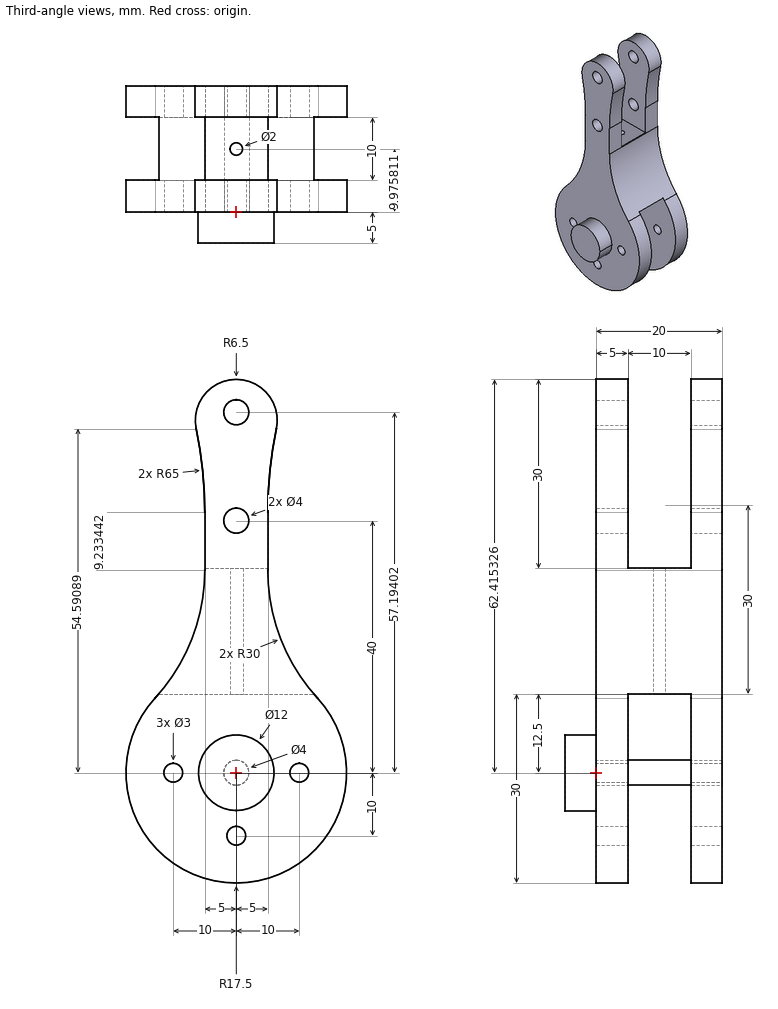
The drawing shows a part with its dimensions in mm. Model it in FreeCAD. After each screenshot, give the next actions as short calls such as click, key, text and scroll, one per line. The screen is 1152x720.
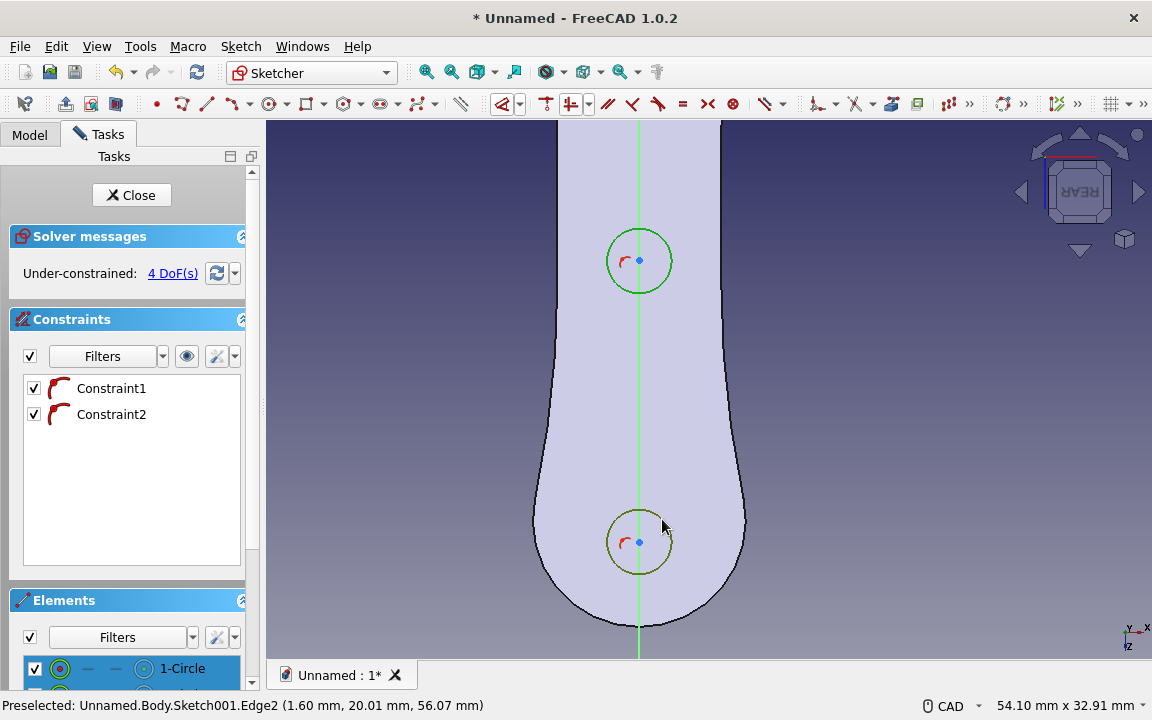
click(683, 104)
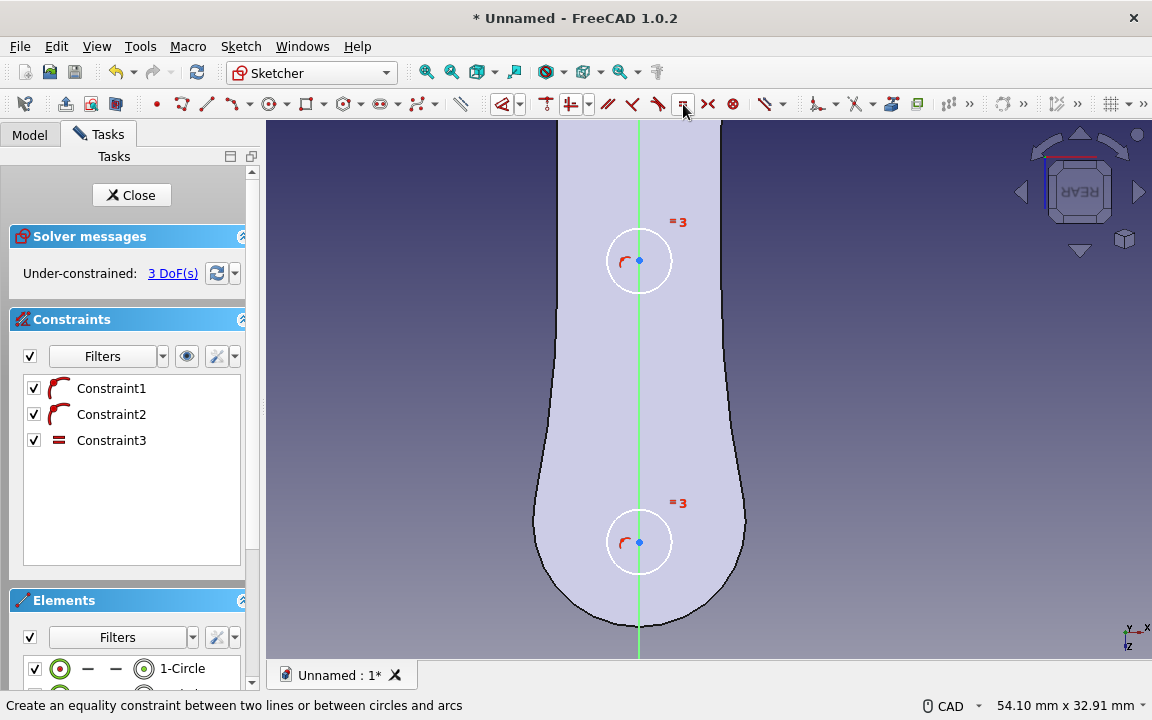
click(662, 238)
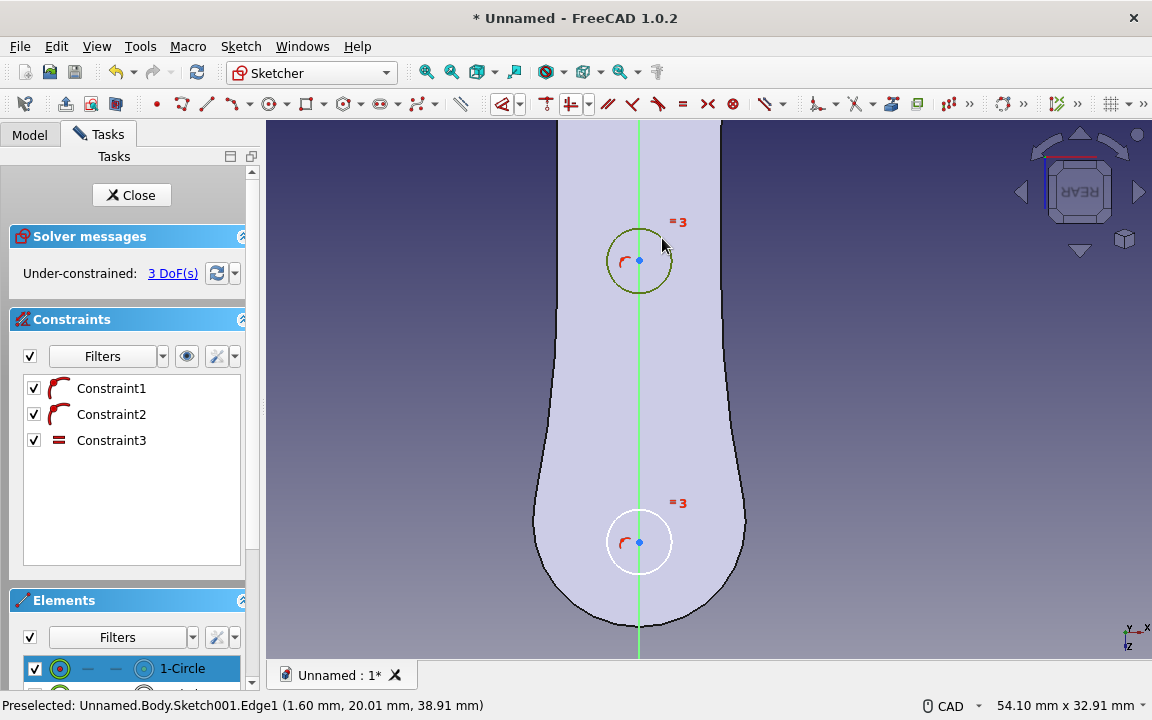
key(k)
key(o)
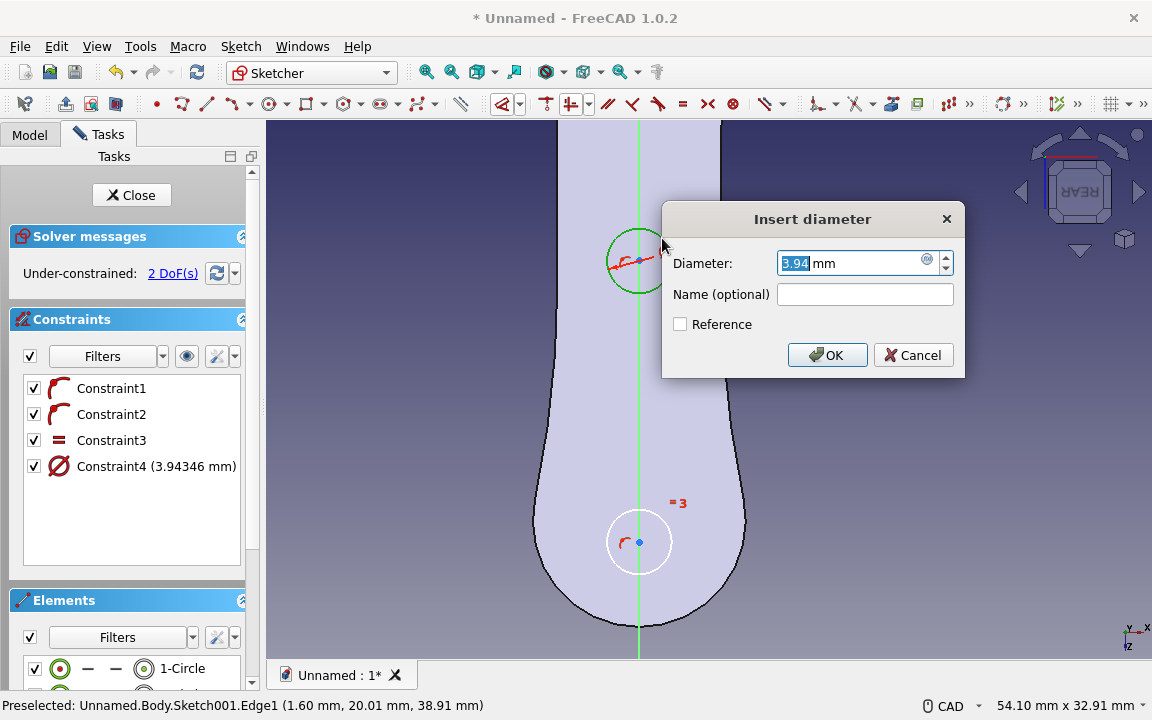
text(4)
key(Return)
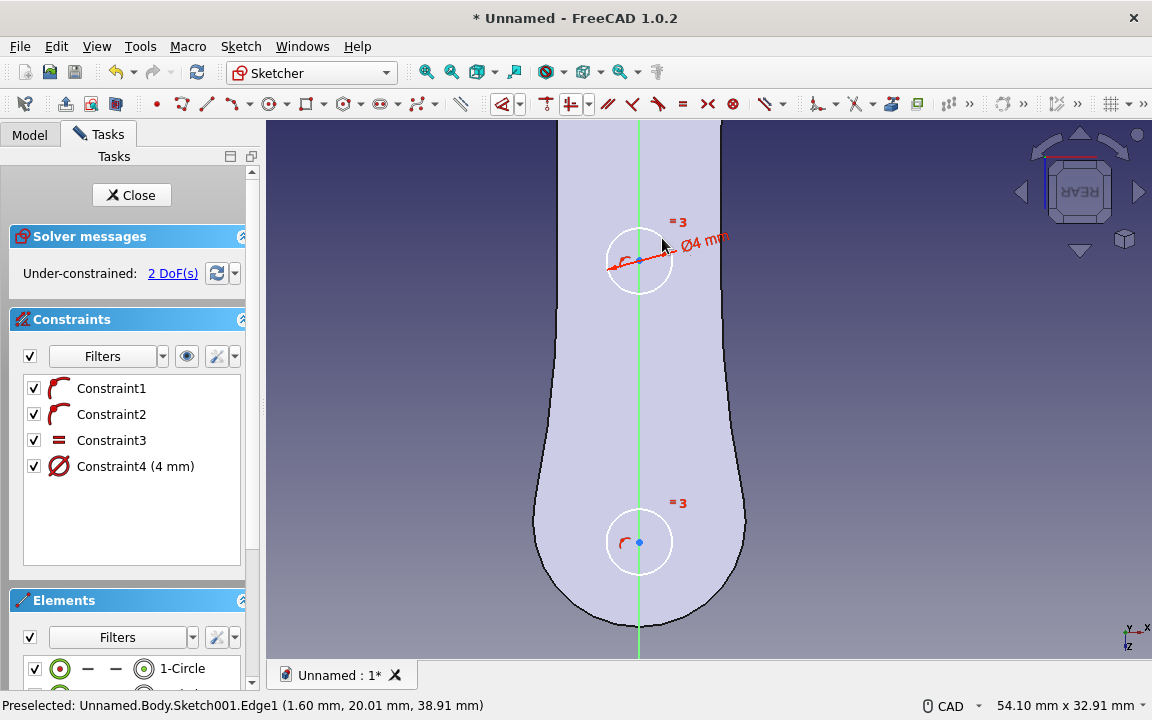
click(639, 261)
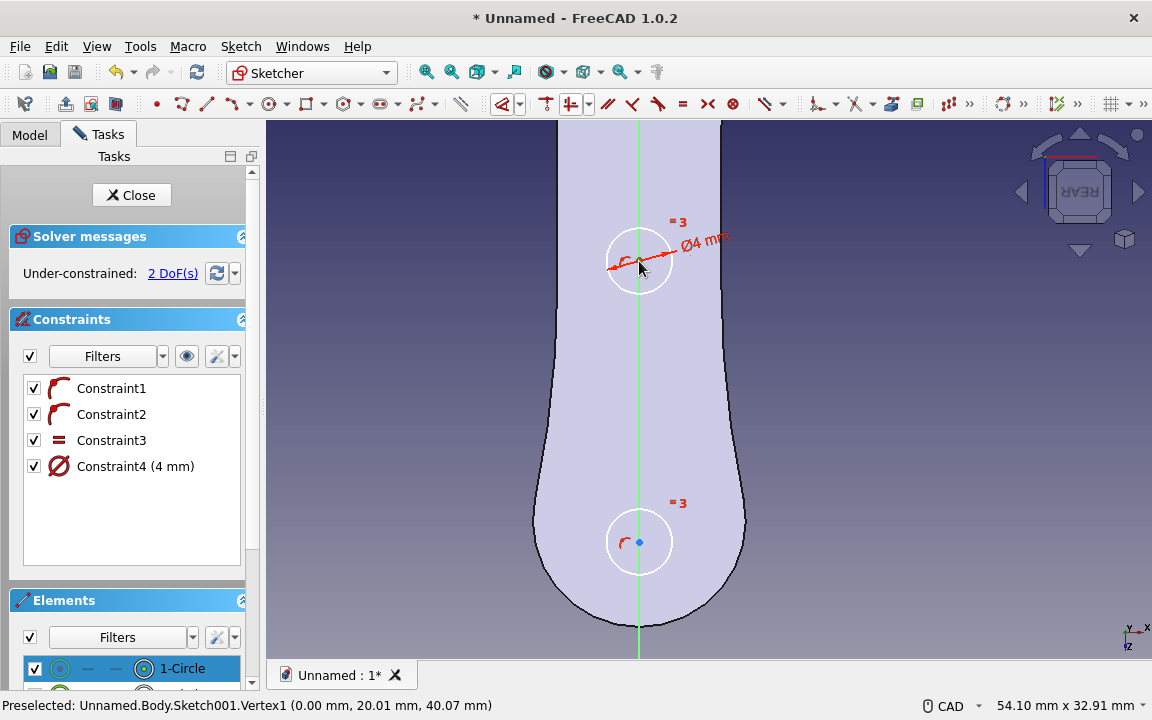
click(520, 104)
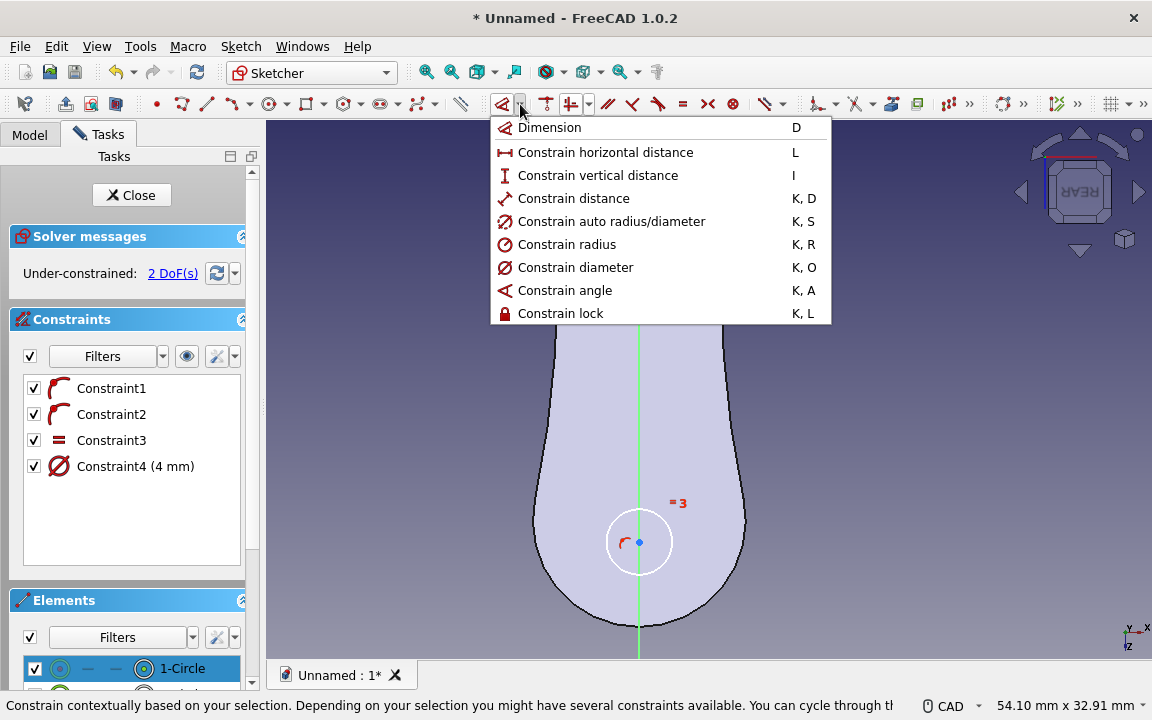
click(661, 176)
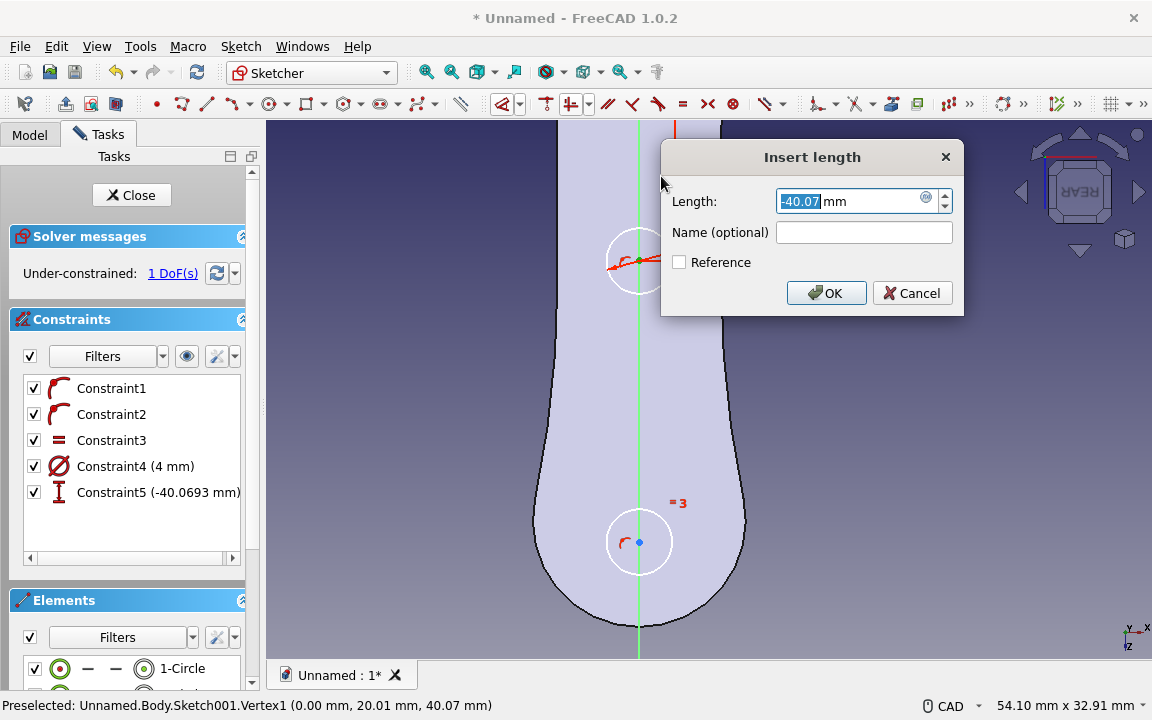
text(-40)
key(Return)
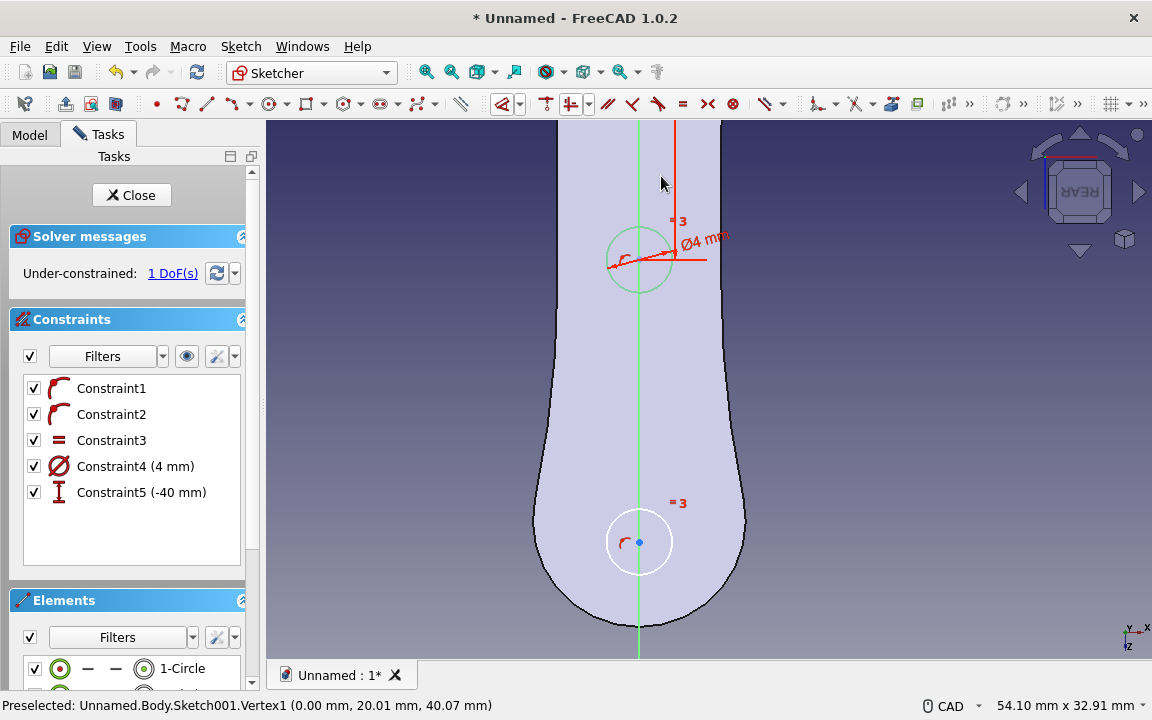
click(639, 542)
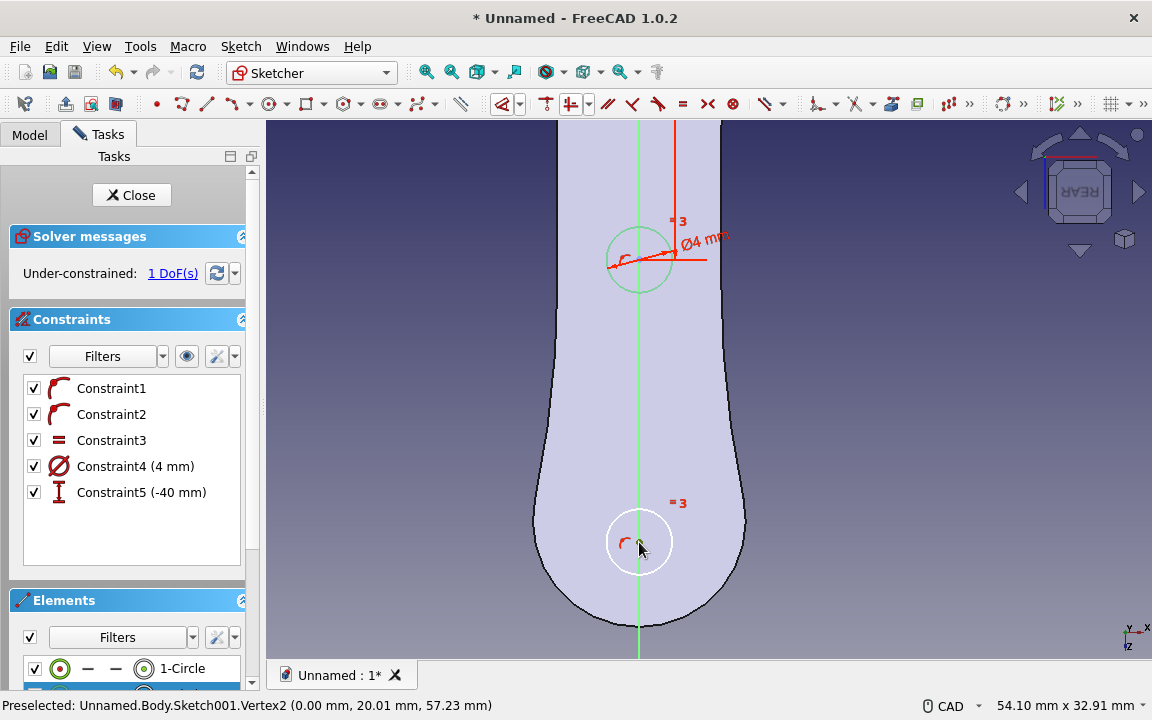
click(520, 104)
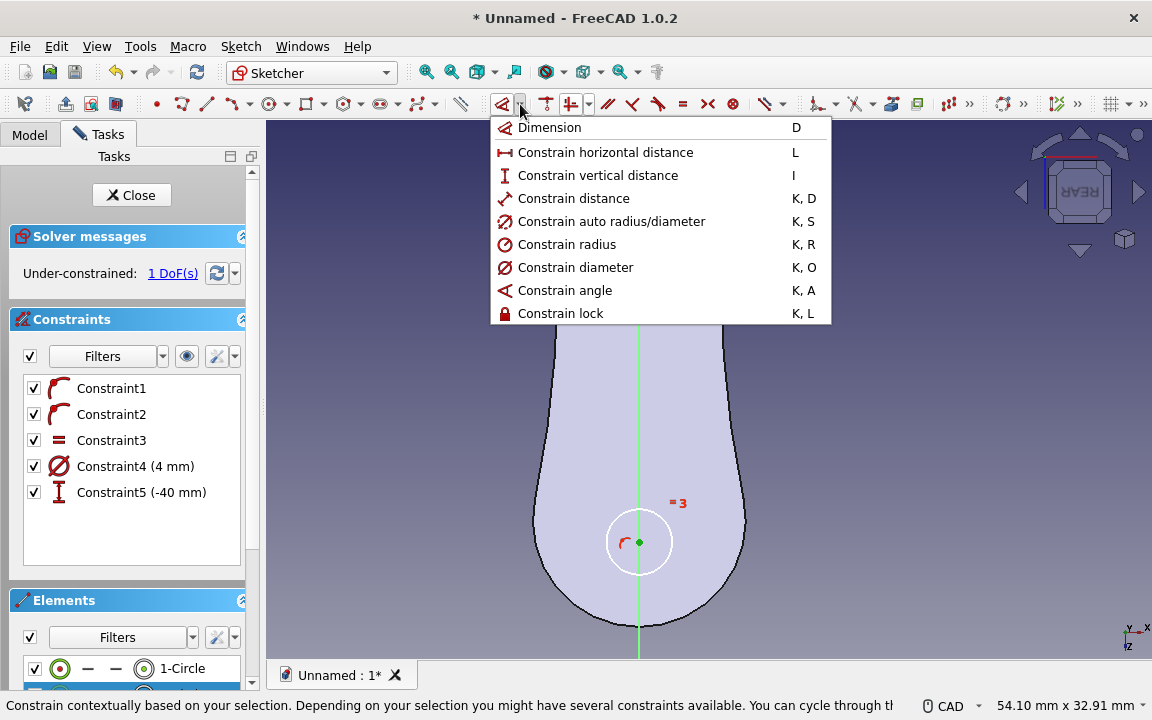
click(661, 176)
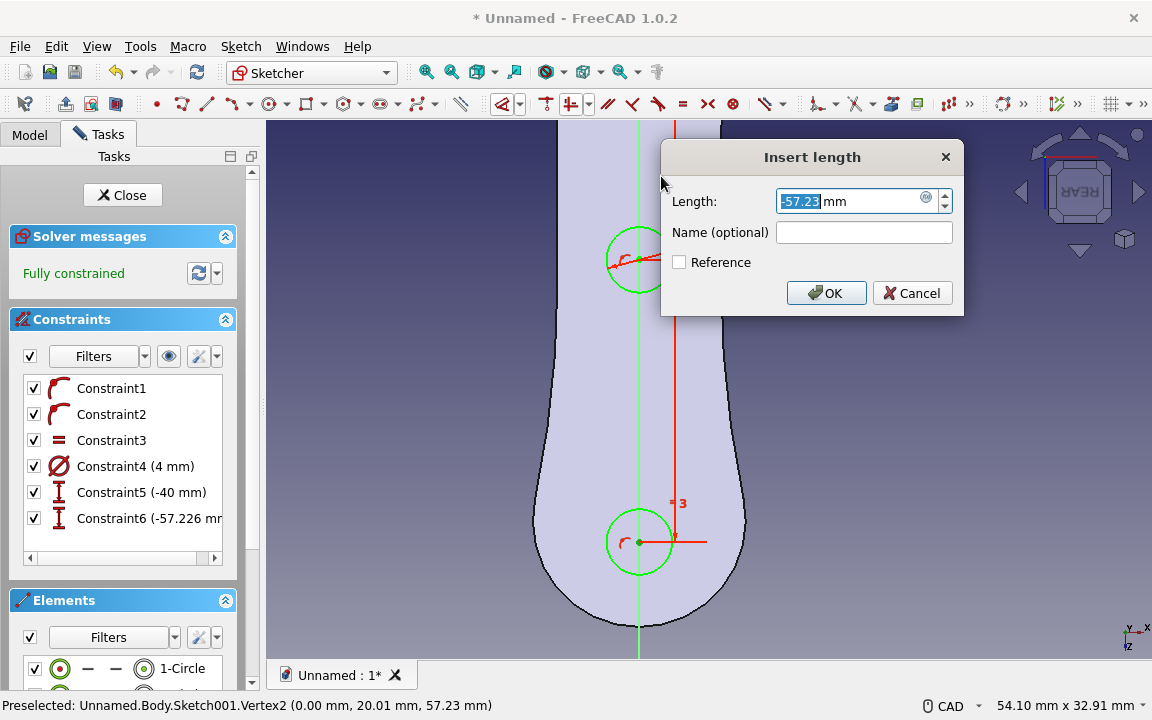
text(-57.19402)
key(Return)